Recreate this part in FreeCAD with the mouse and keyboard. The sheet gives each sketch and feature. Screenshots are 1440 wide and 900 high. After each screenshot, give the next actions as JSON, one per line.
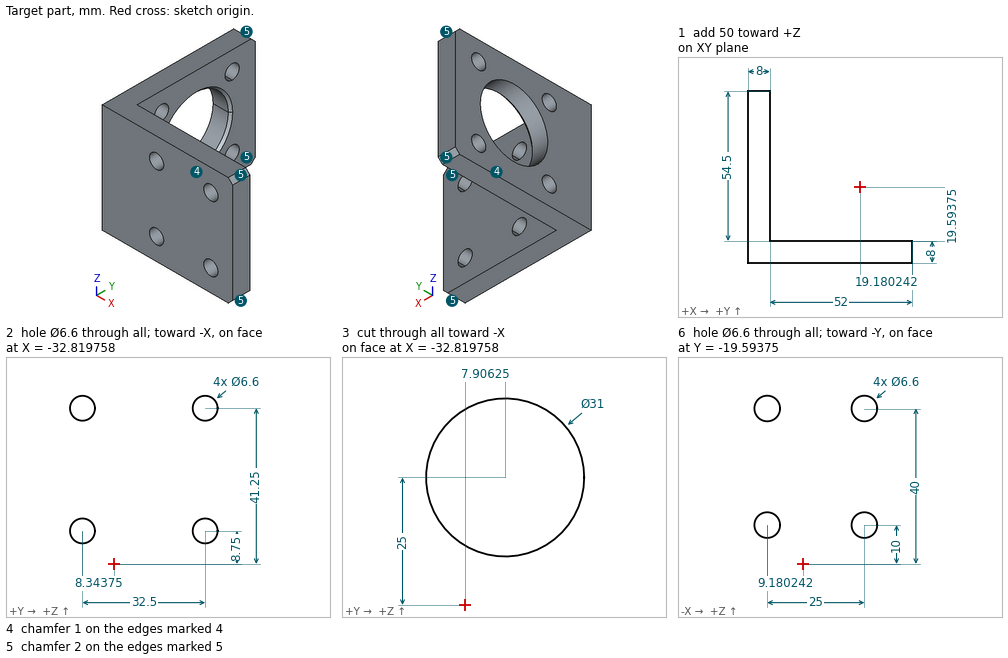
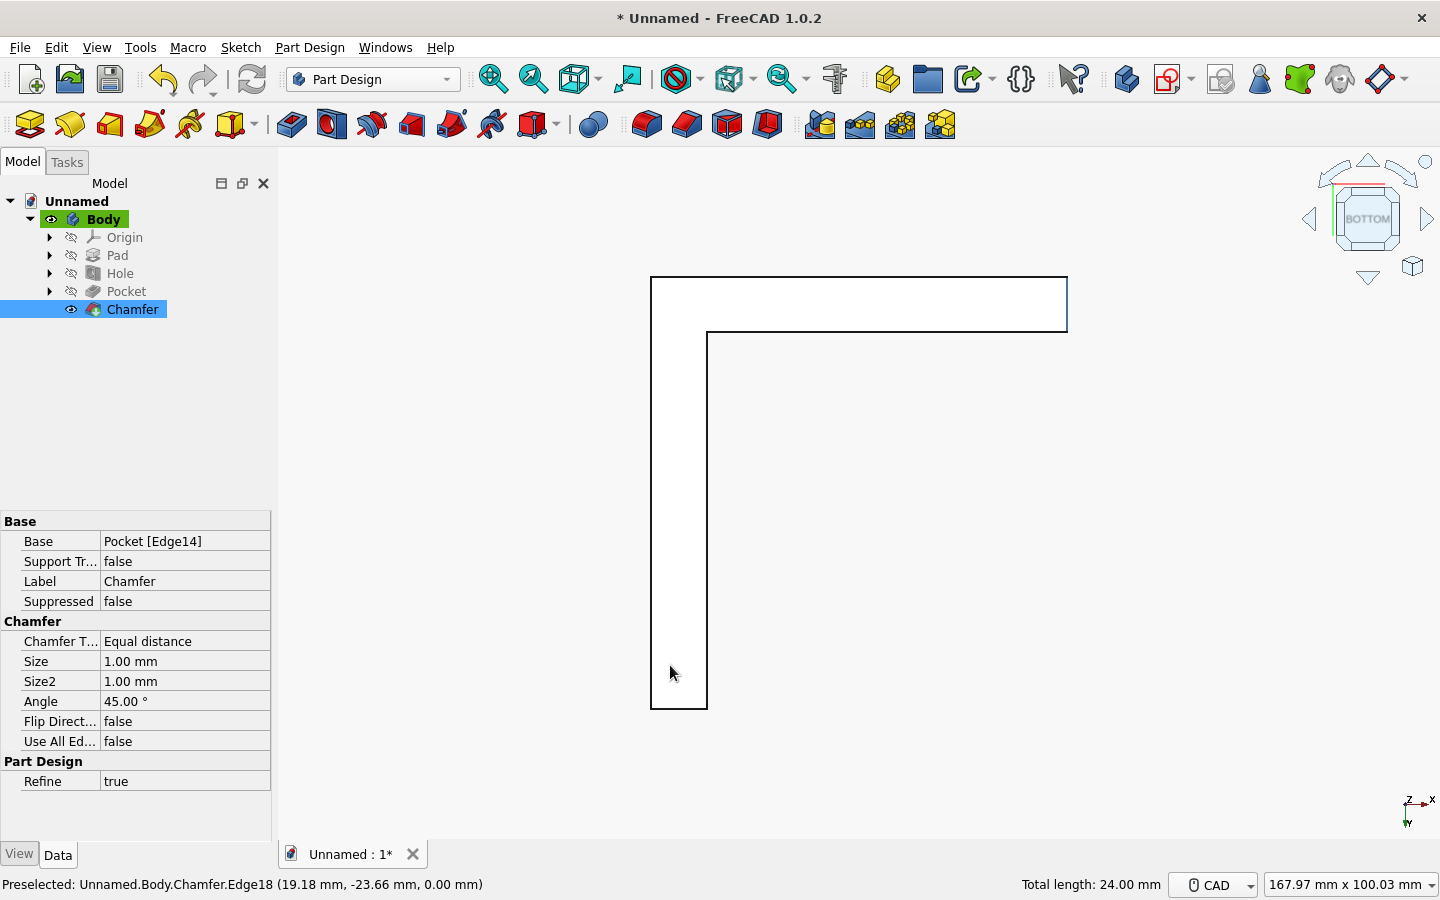
{"action": "left_click", "coordinate": [679, 708], "text": "ctrl"}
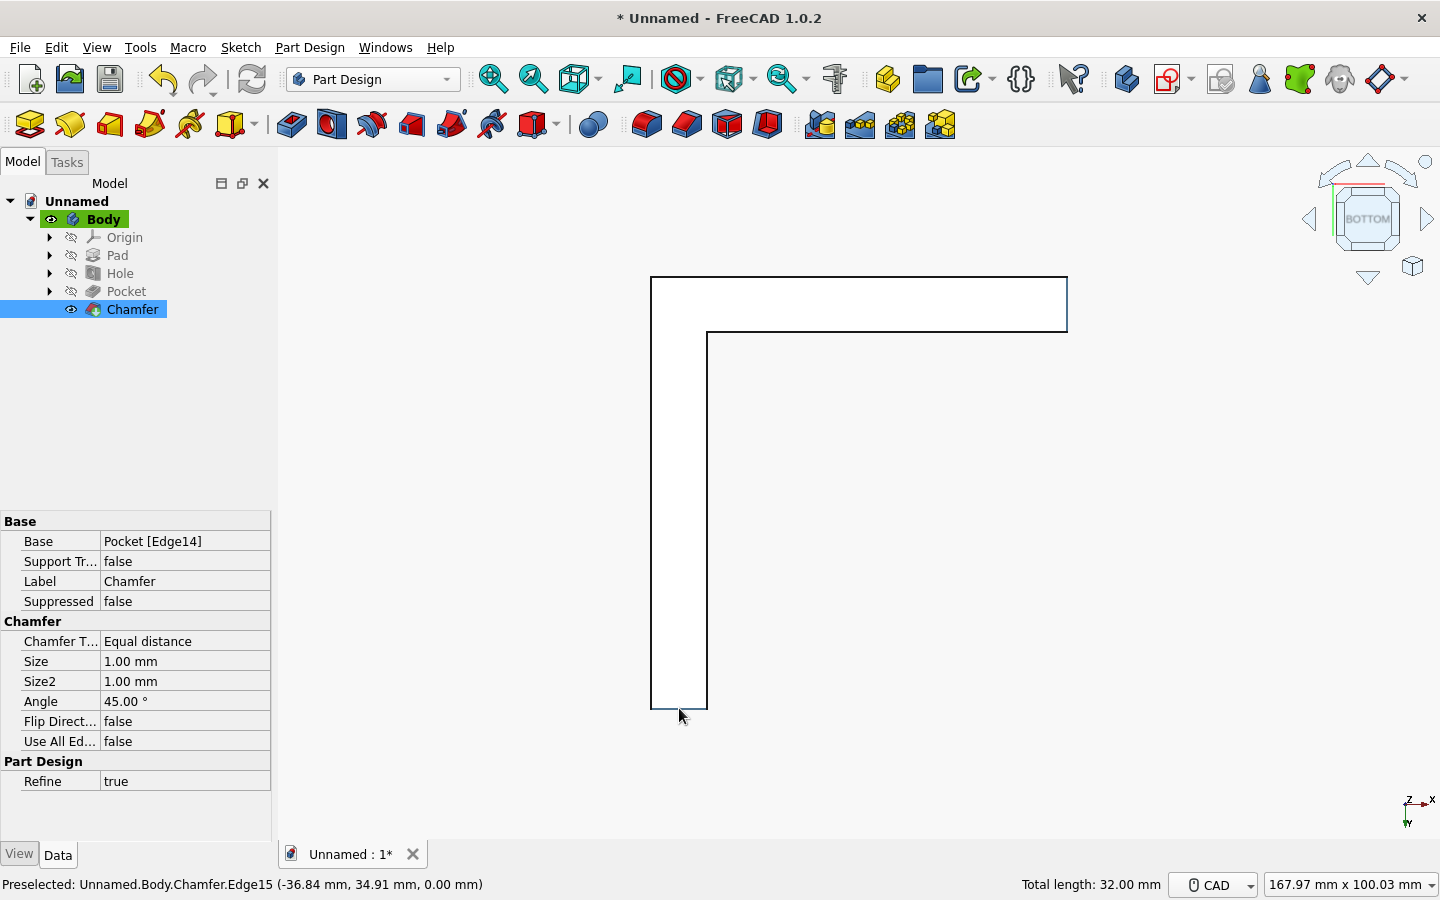
{"action": "left_click", "coordinate": [688, 124]}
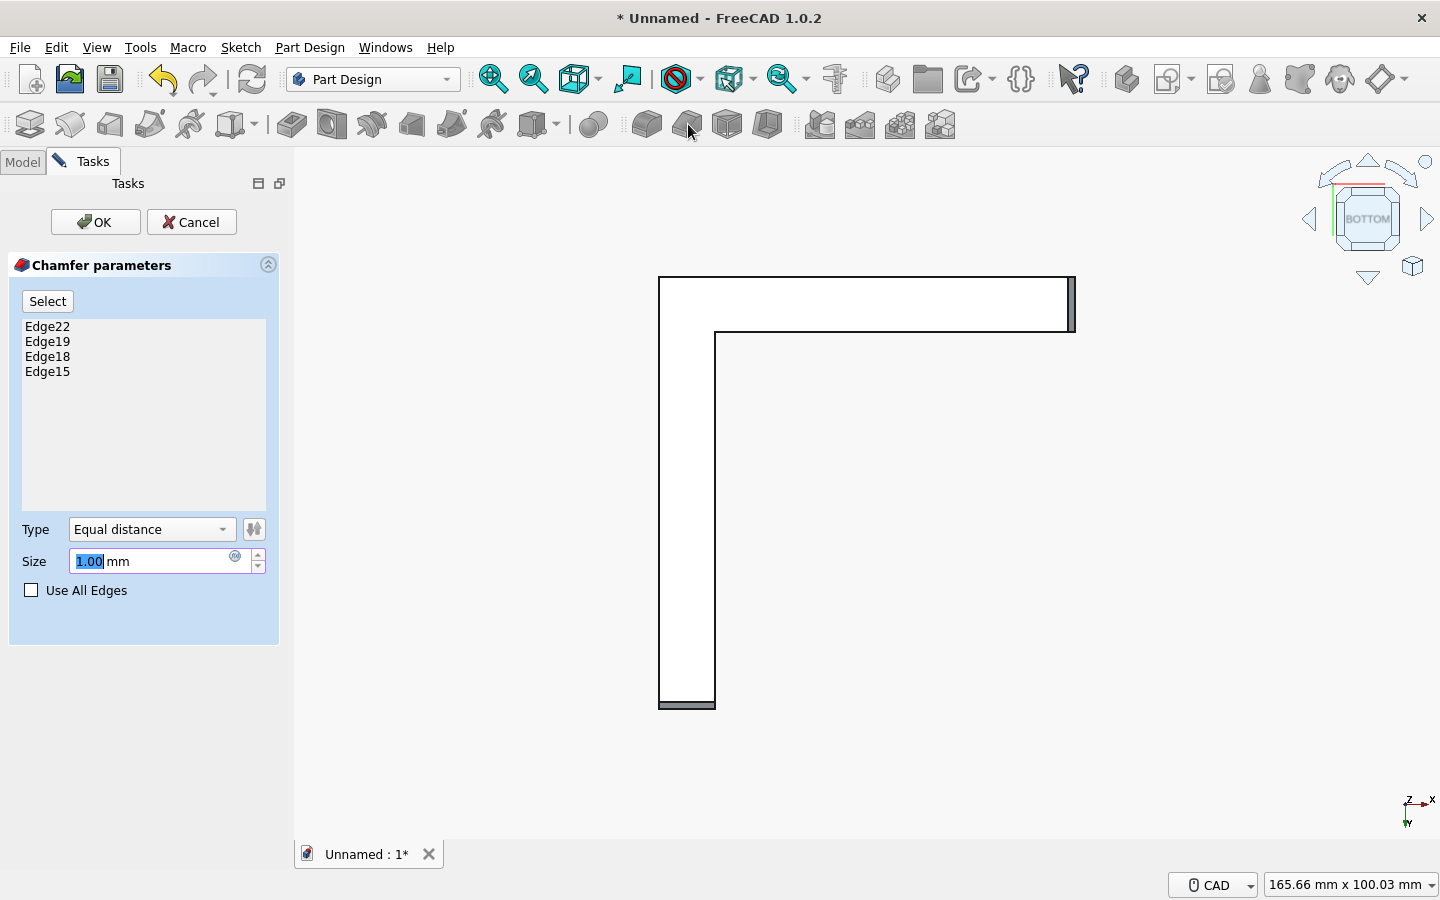
{"action": "type", "text": "2"}
{"action": "key", "text": "Tab"}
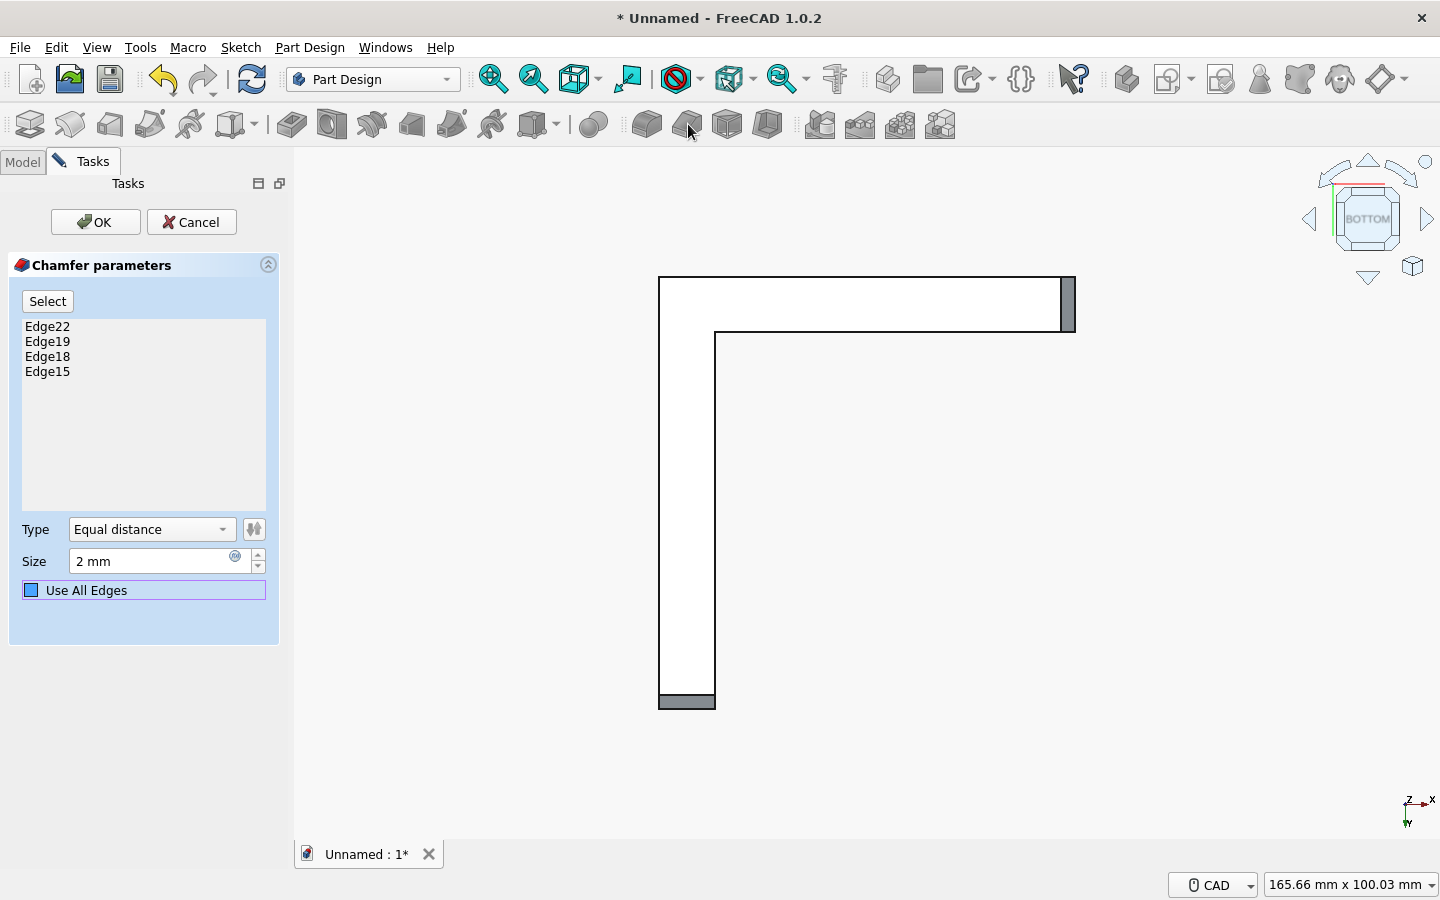
{"action": "left_click", "coordinate": [96, 222]}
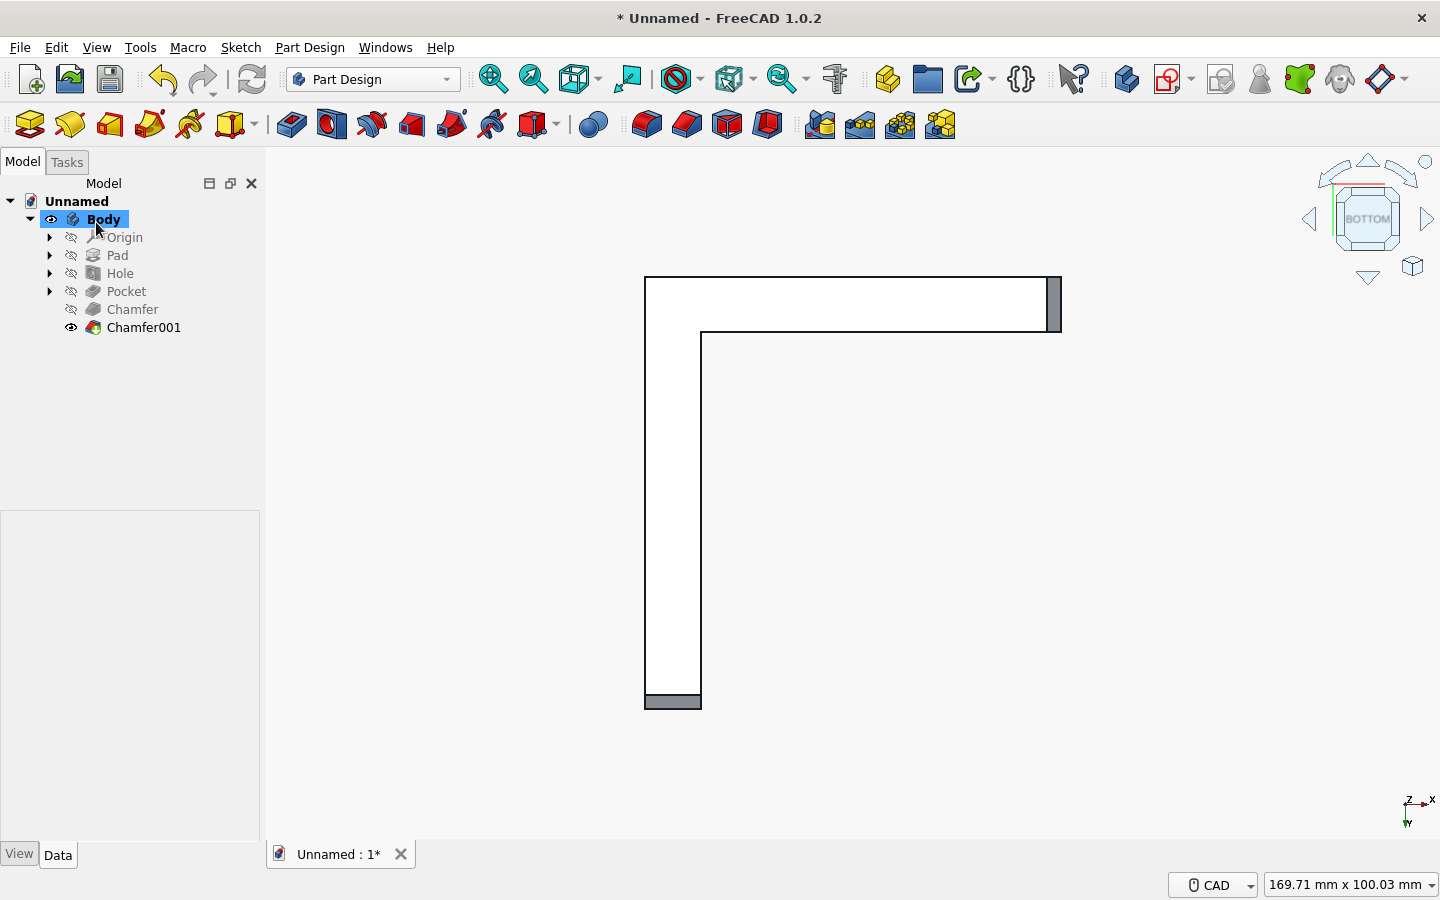
{"action": "key", "text": "4"}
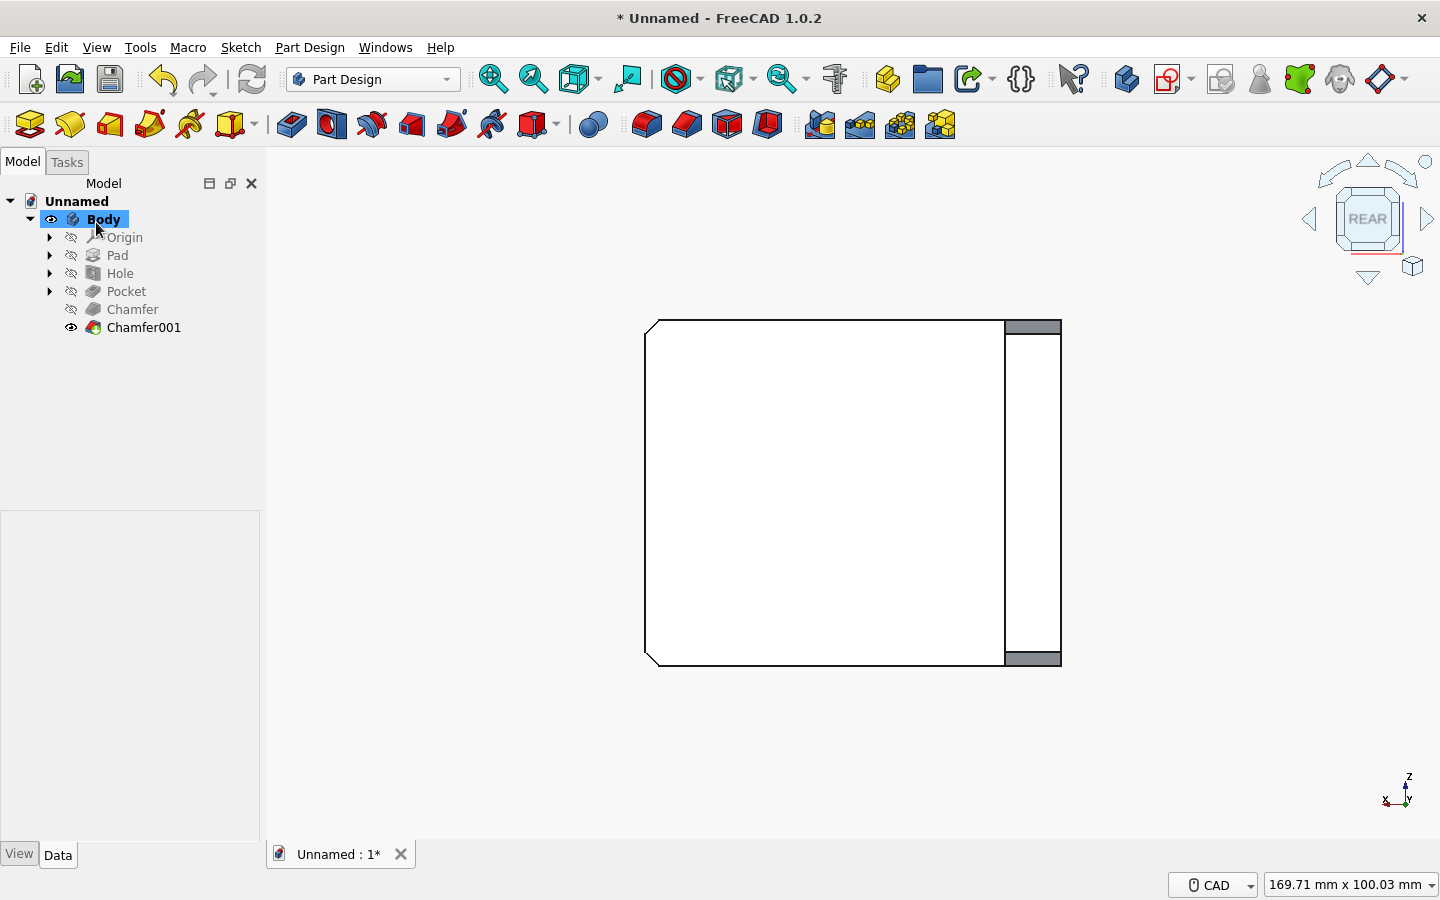
{"action": "left_click", "coordinate": [825, 492]}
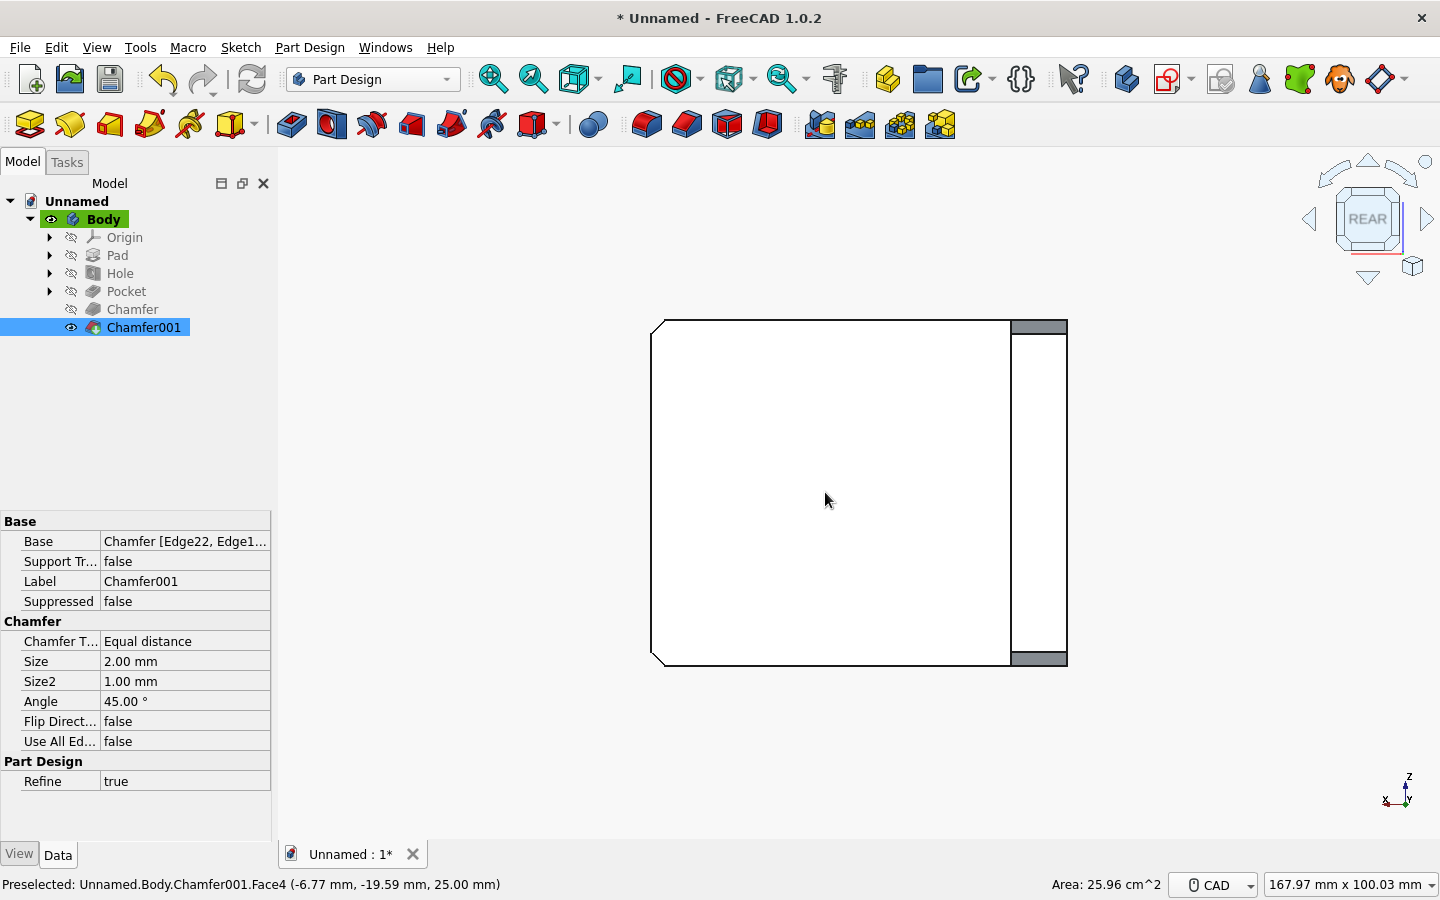
{"action": "left_click", "coordinate": [1168, 80]}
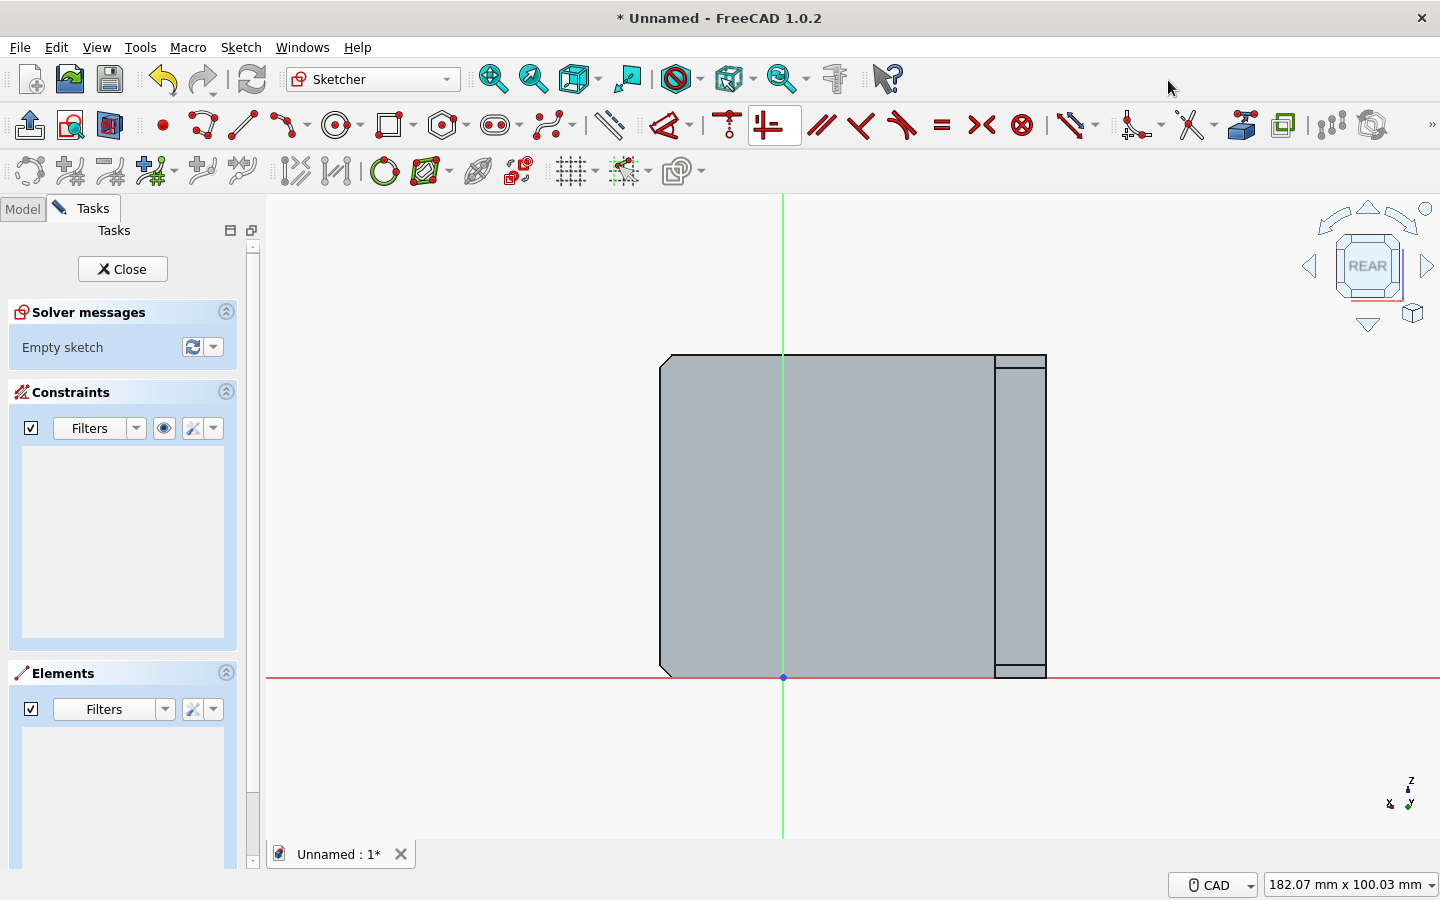
{"action": "scroll", "coordinate": [846, 582], "scroll_direction": "up", "scroll_amount": 2}